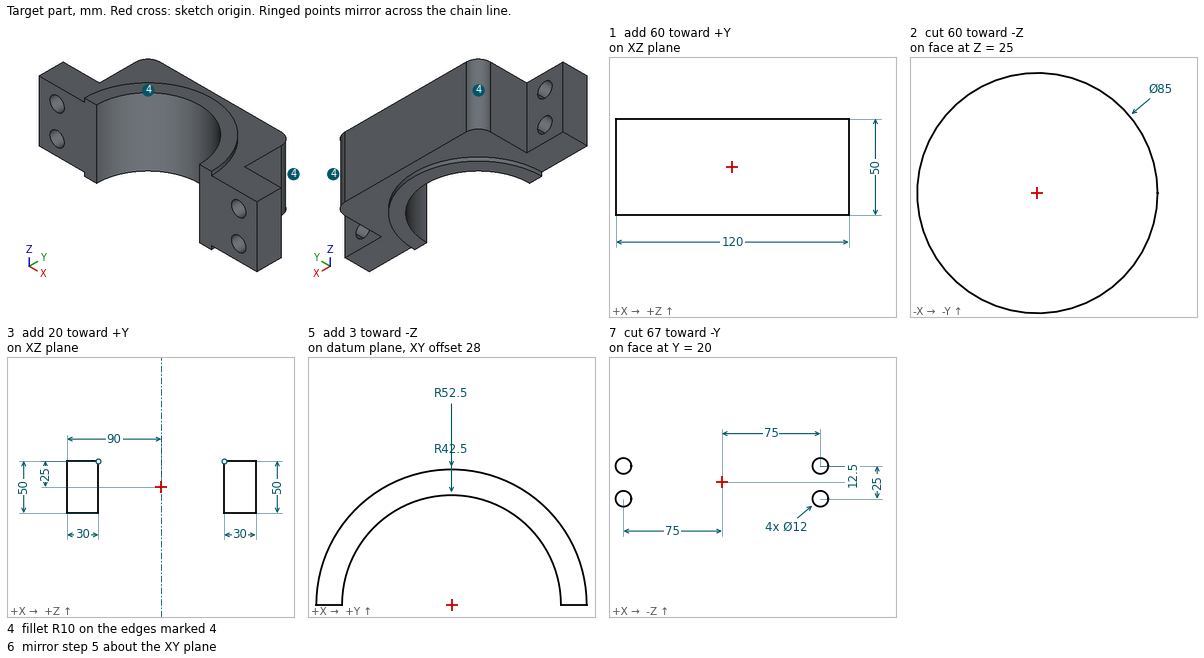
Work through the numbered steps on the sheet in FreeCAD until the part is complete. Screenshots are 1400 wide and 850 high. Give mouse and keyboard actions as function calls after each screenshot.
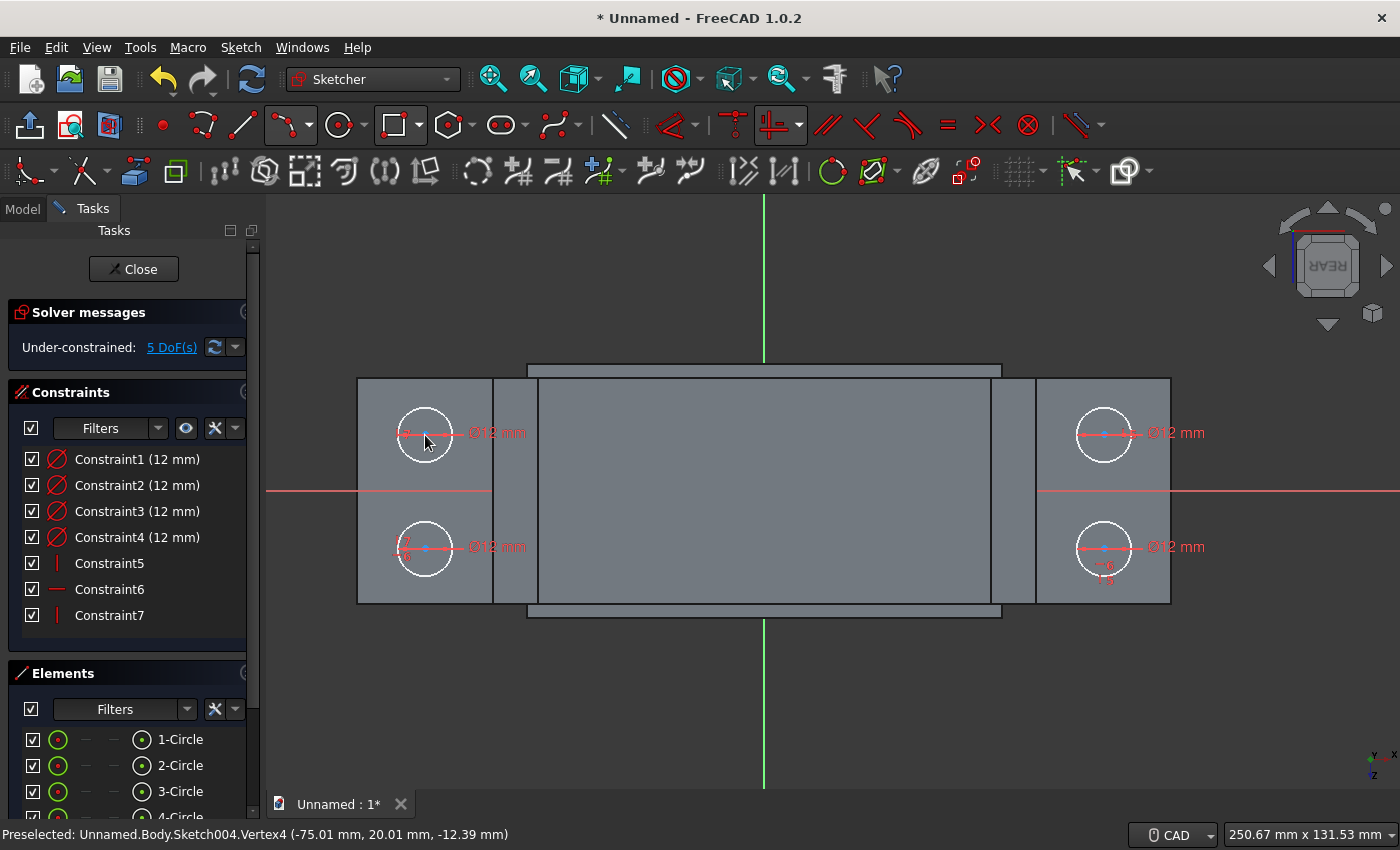
click(1104, 435)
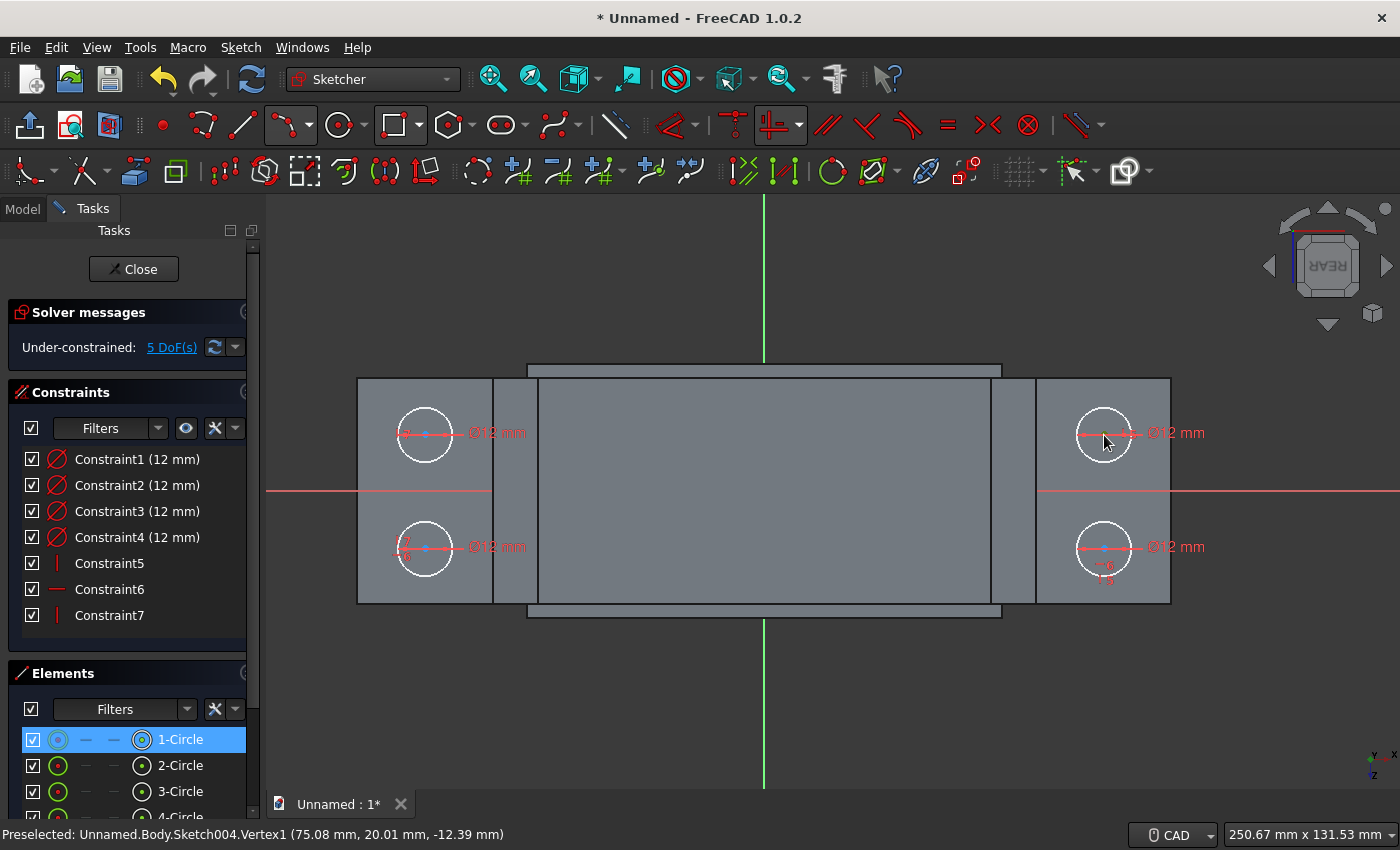
click(425, 435)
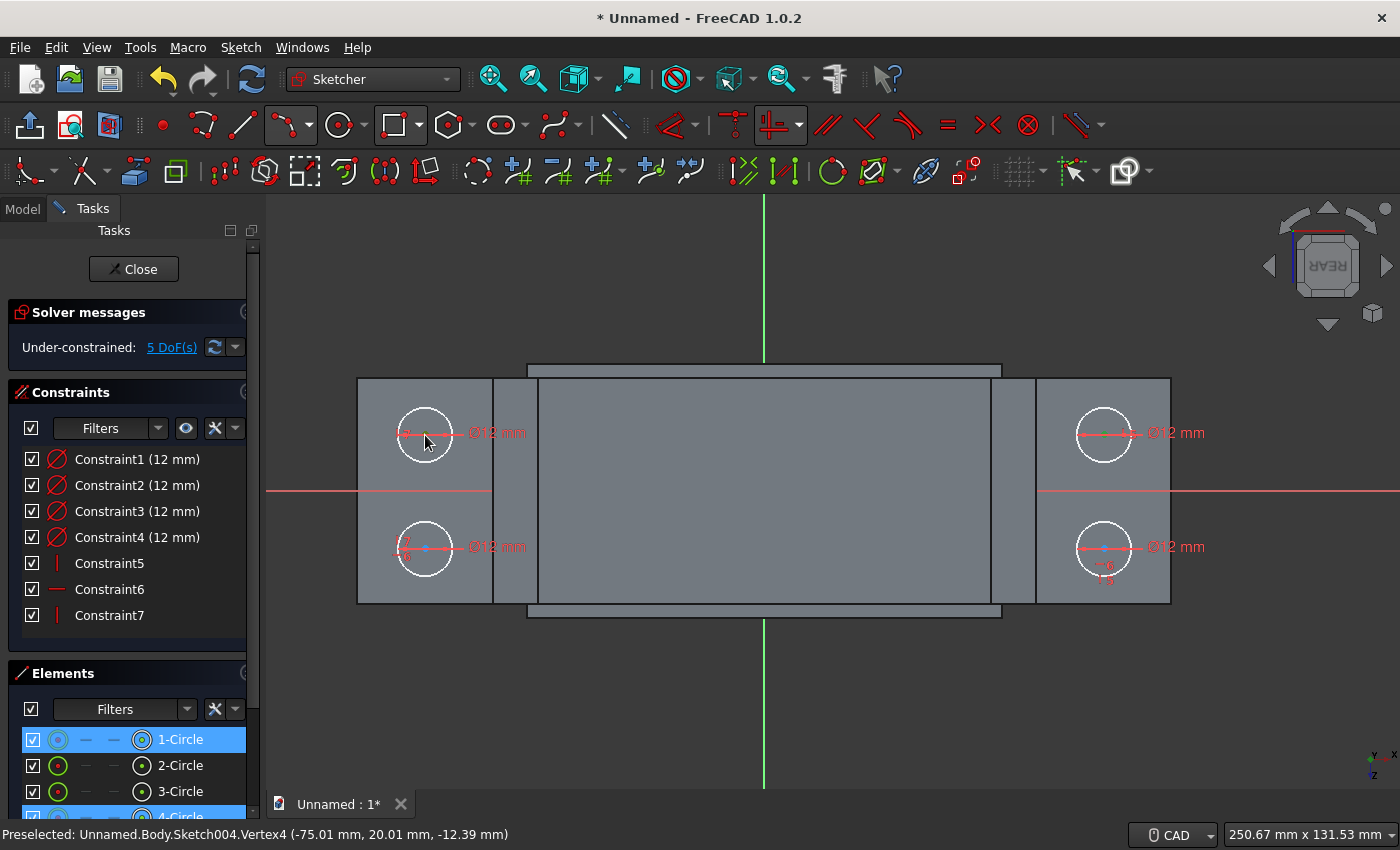
click(802, 126)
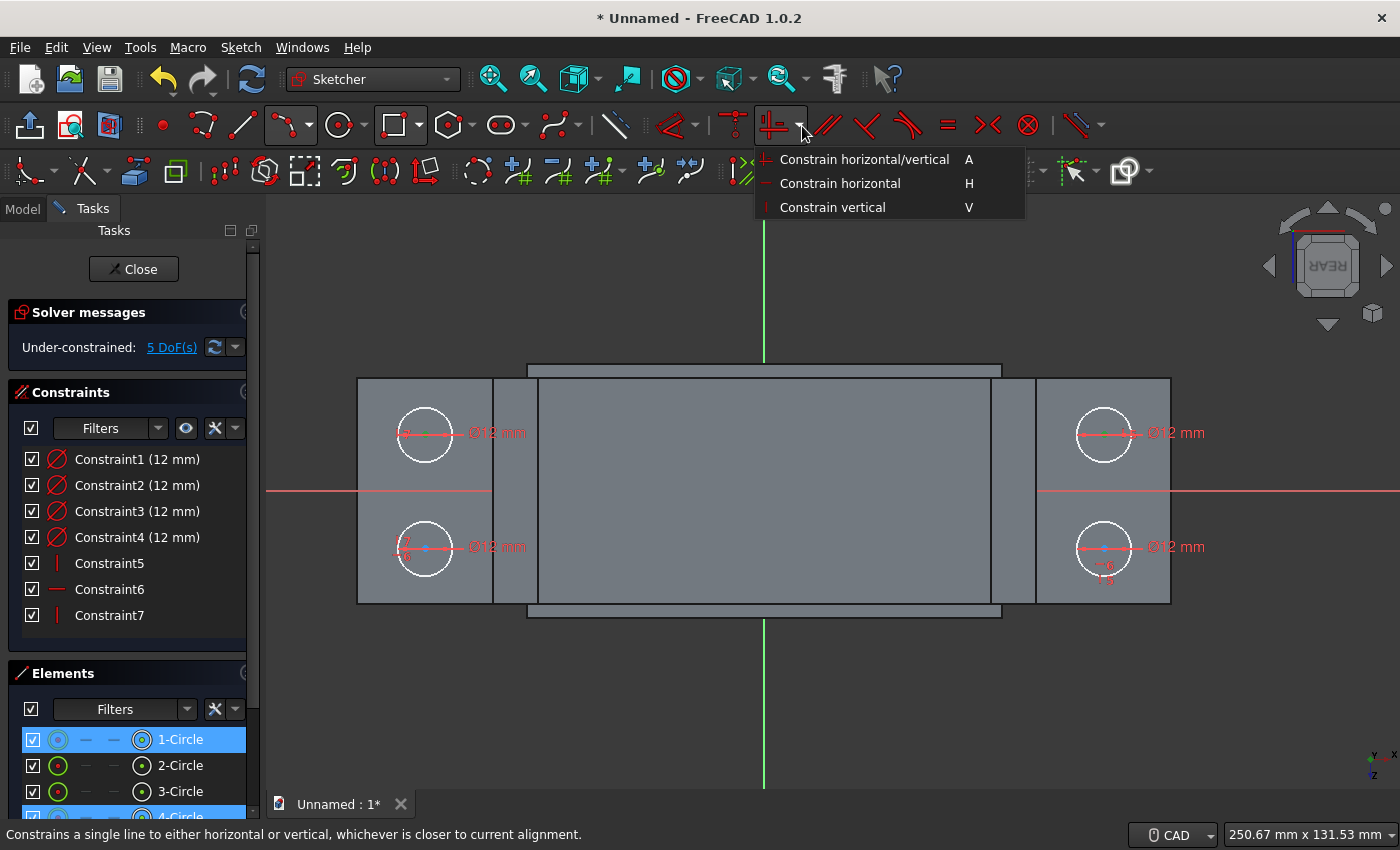
click(890, 183)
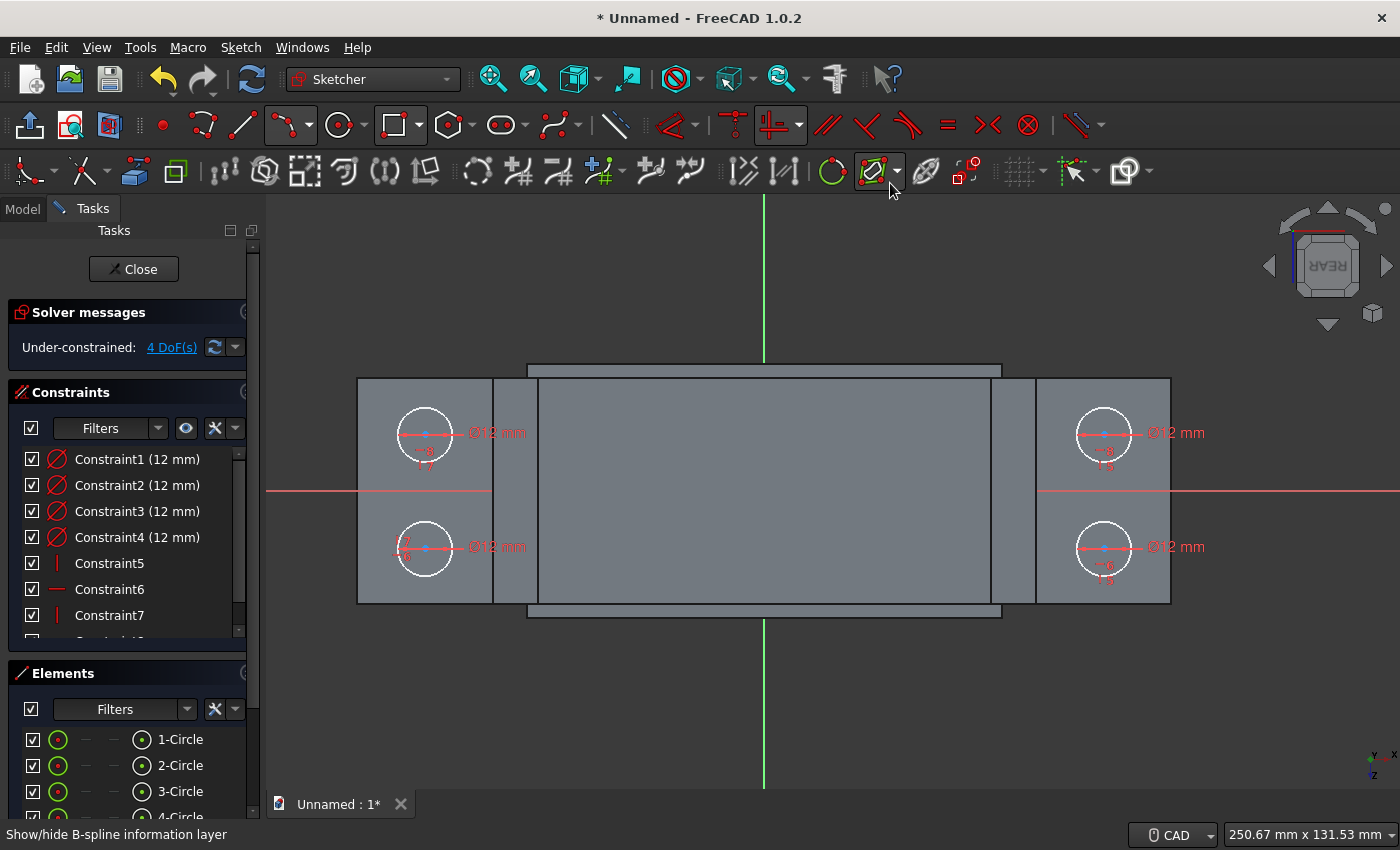
click(670, 126)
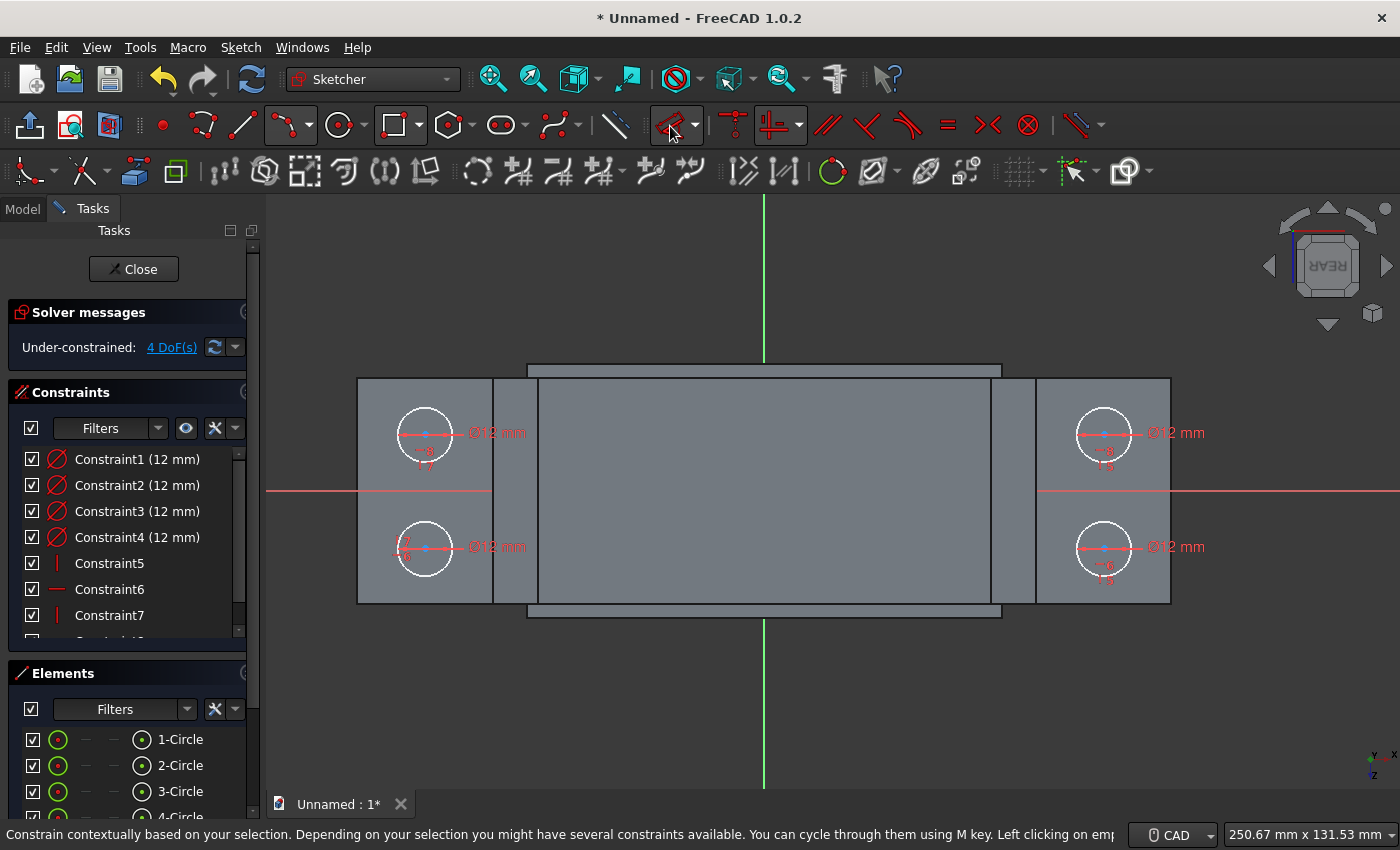
click(1104, 435)
click(934, 401)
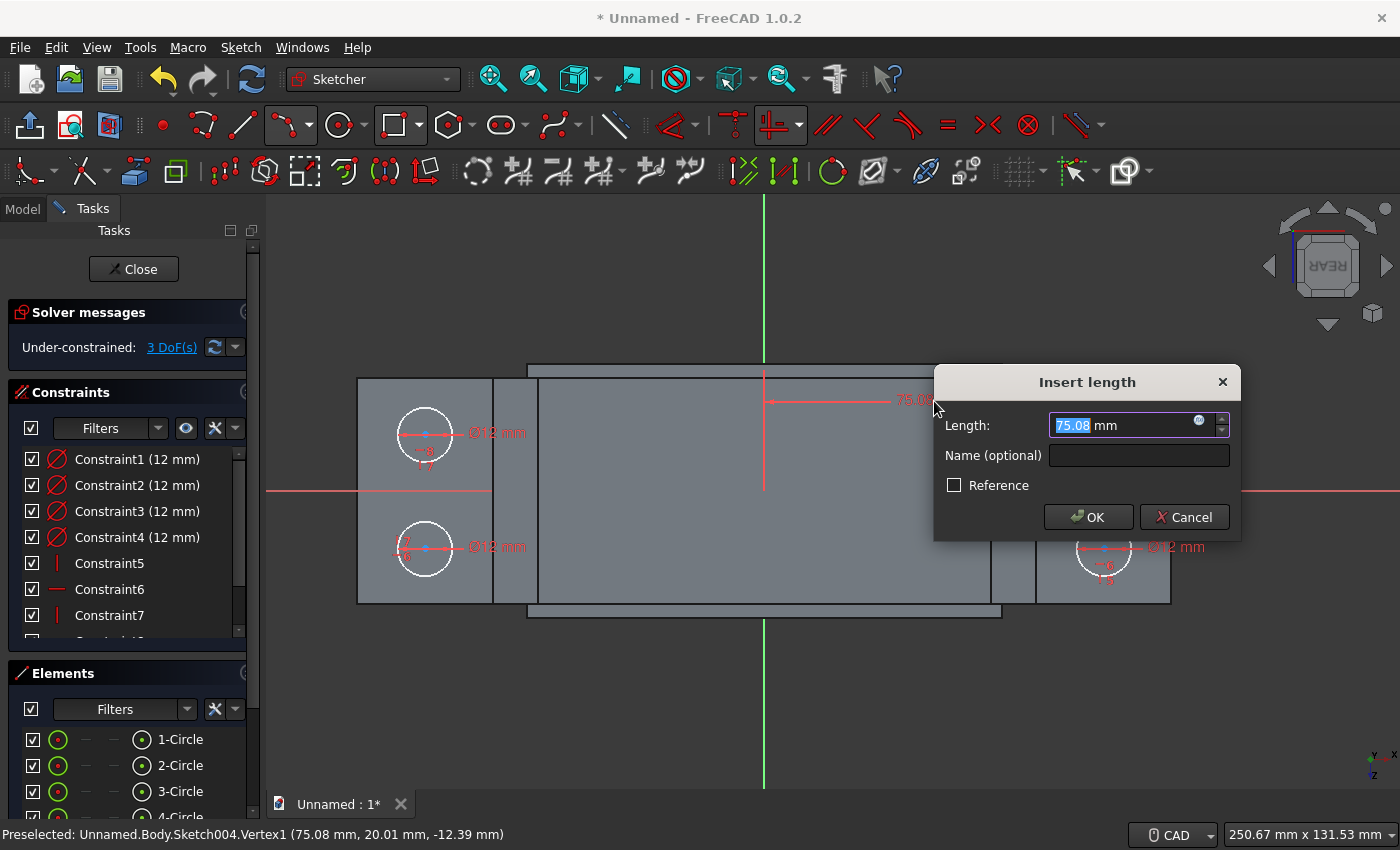
text(75)
key(Return)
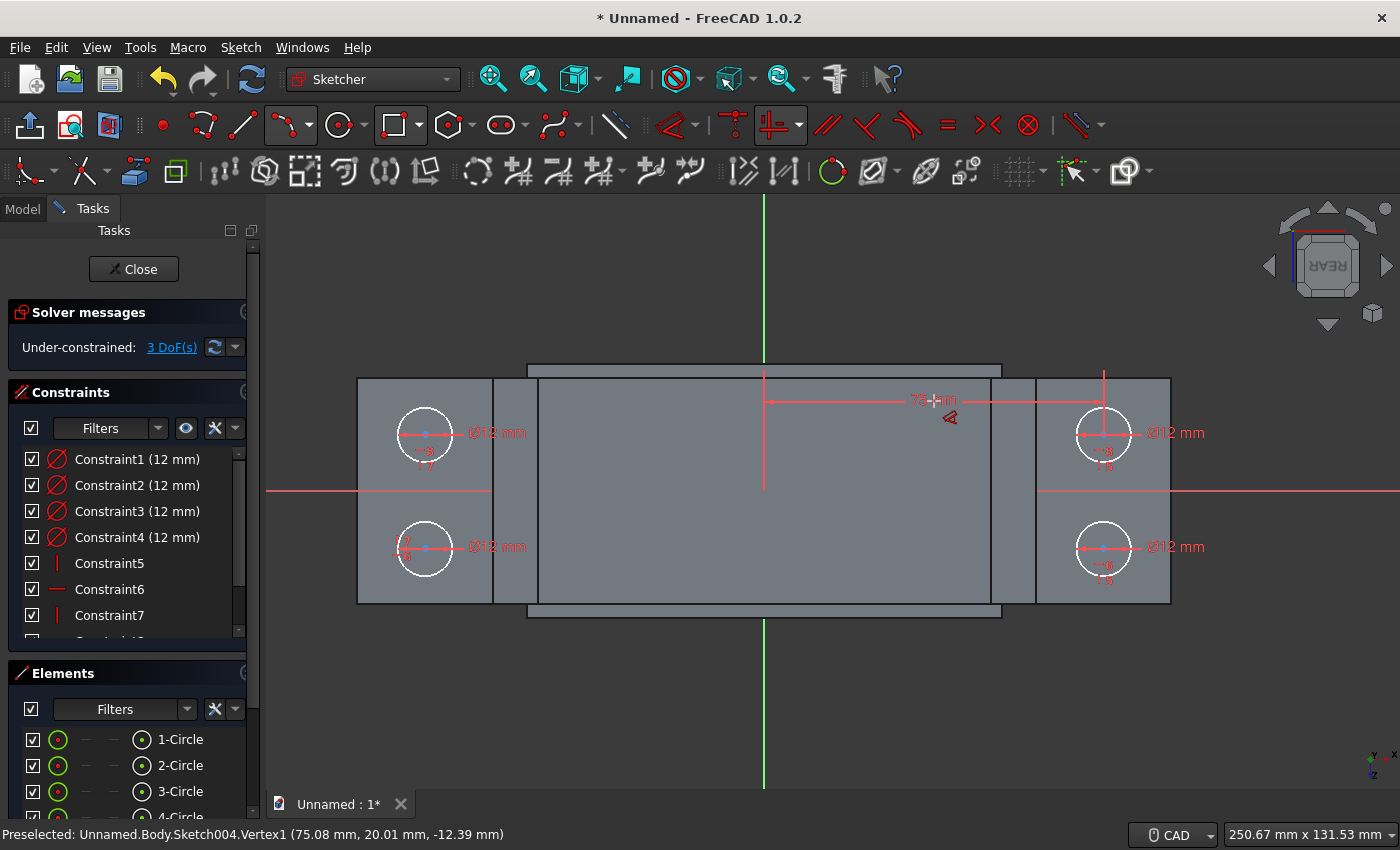
click(425, 549)
click(595, 583)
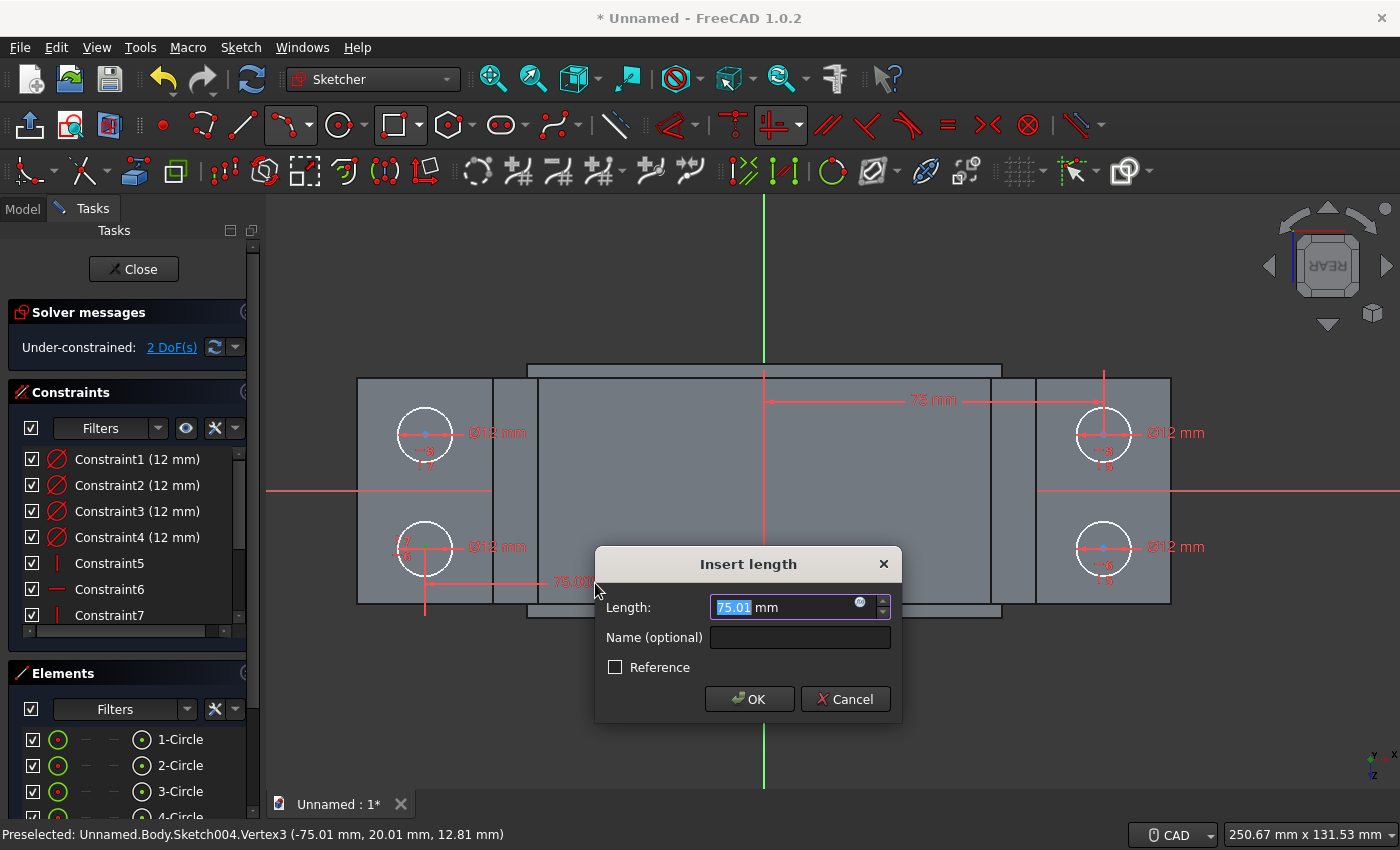
text(75)
key(Return)